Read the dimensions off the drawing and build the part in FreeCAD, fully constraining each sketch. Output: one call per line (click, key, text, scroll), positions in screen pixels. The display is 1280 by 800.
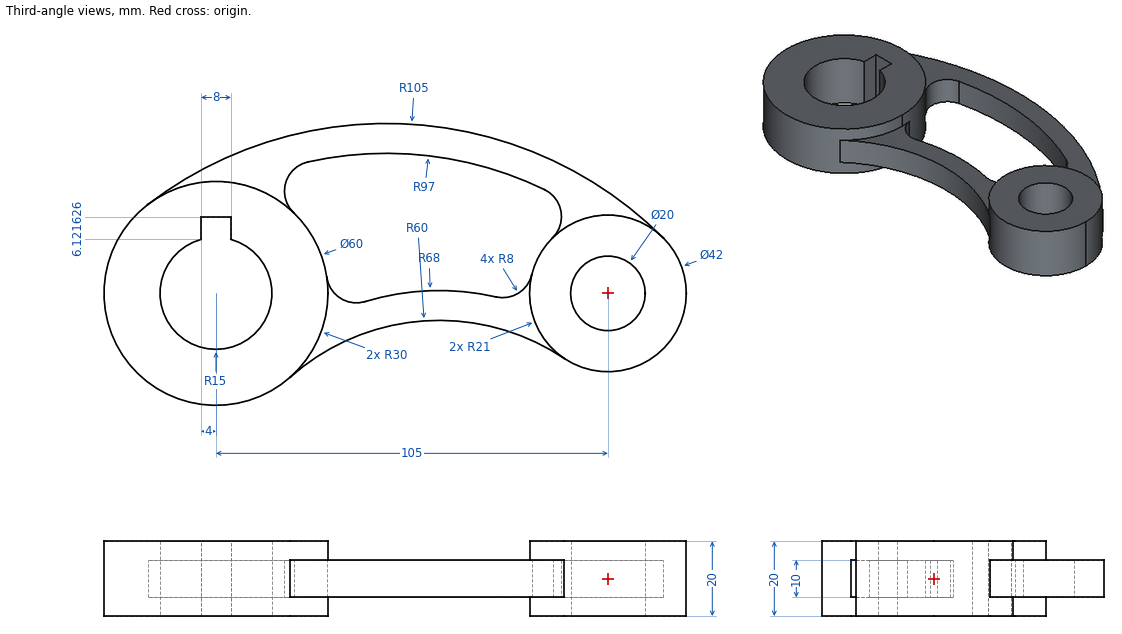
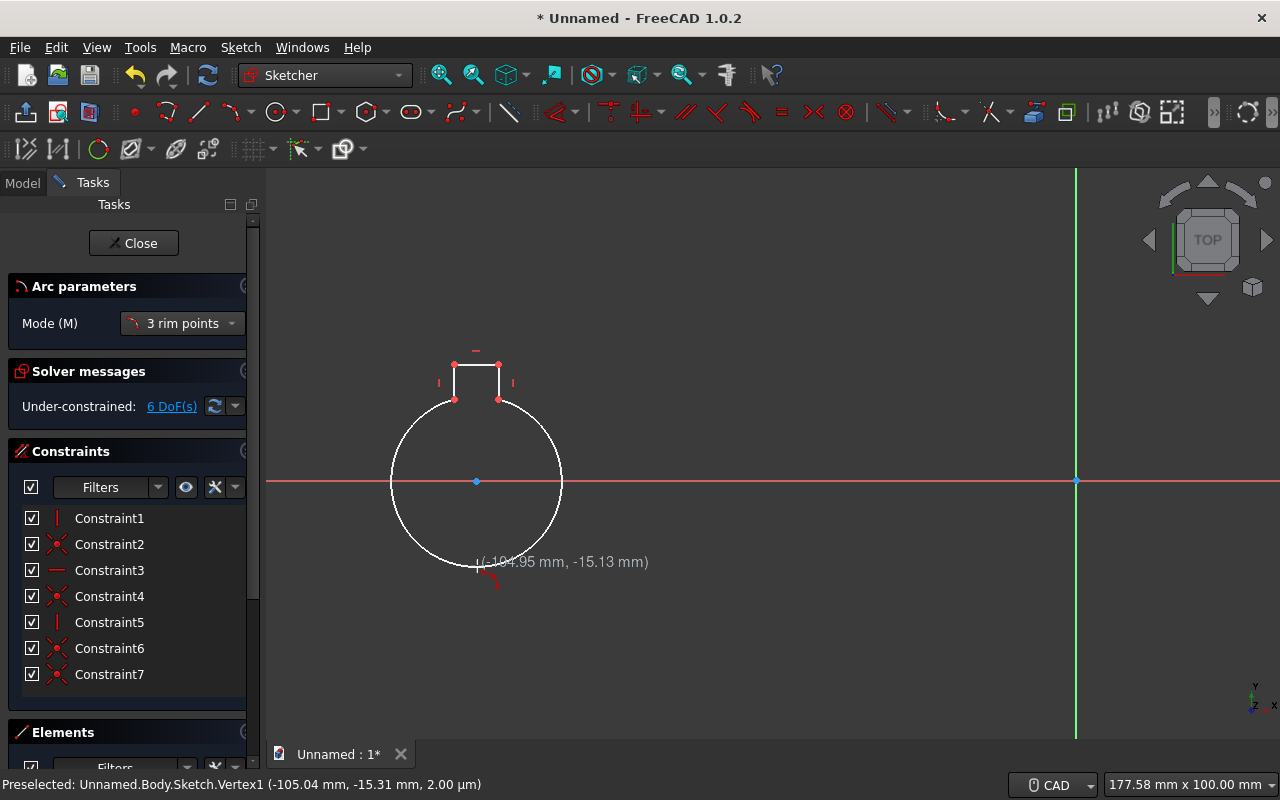
key(g)
key(c)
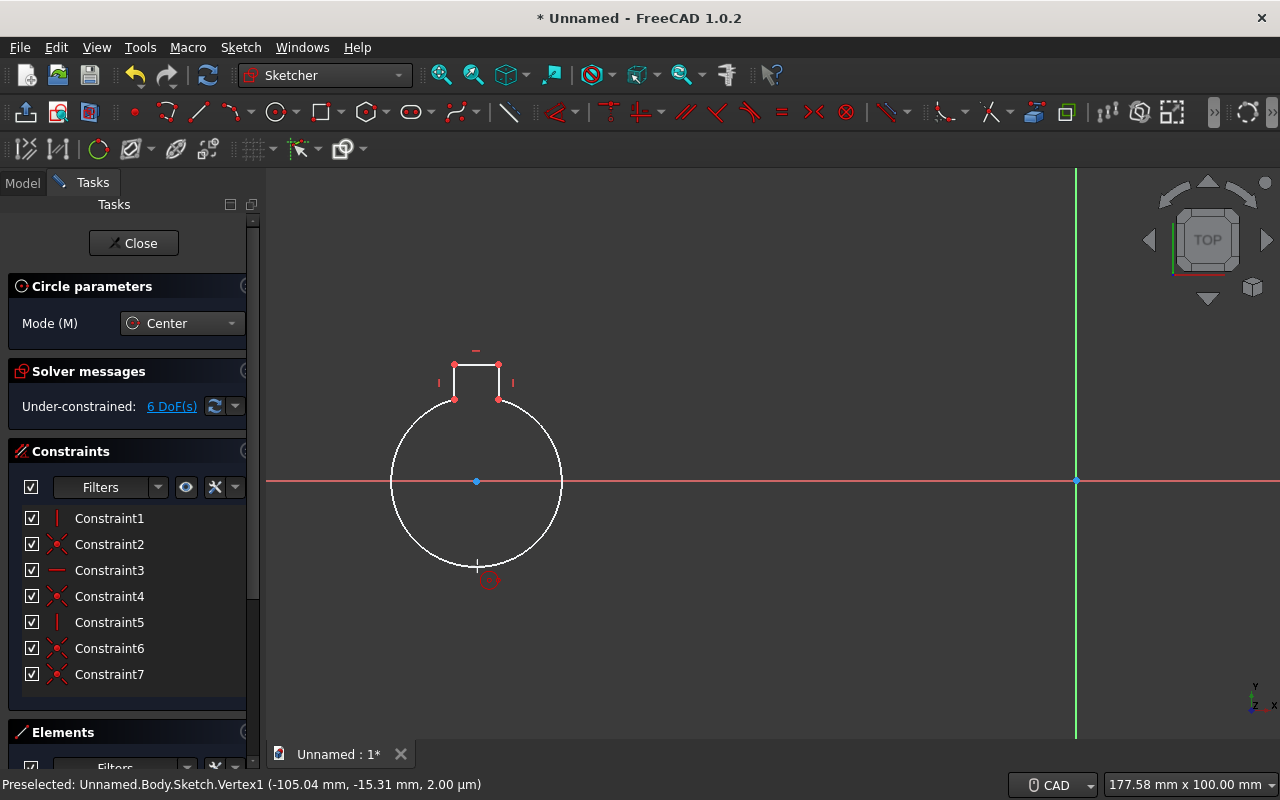
click(477, 481)
move(598, 359)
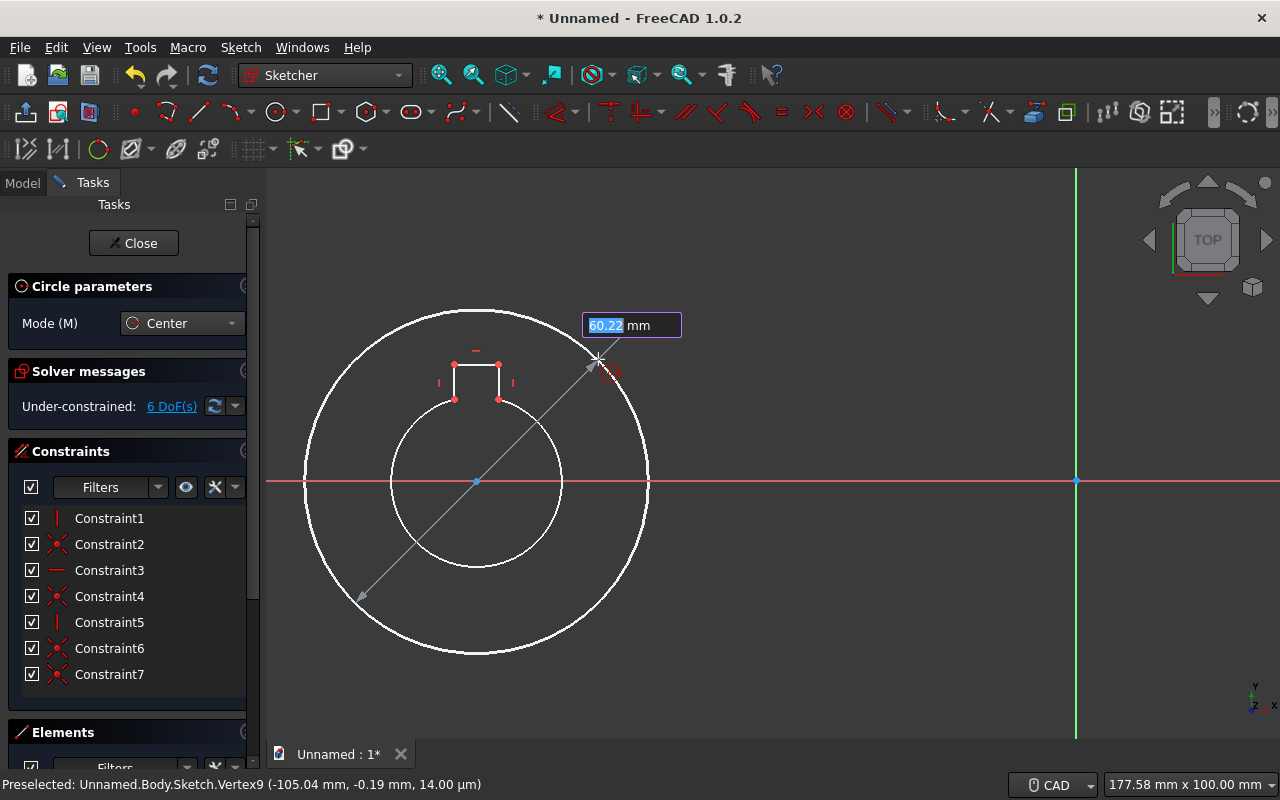
text(60)
key(Return)
key(Escape)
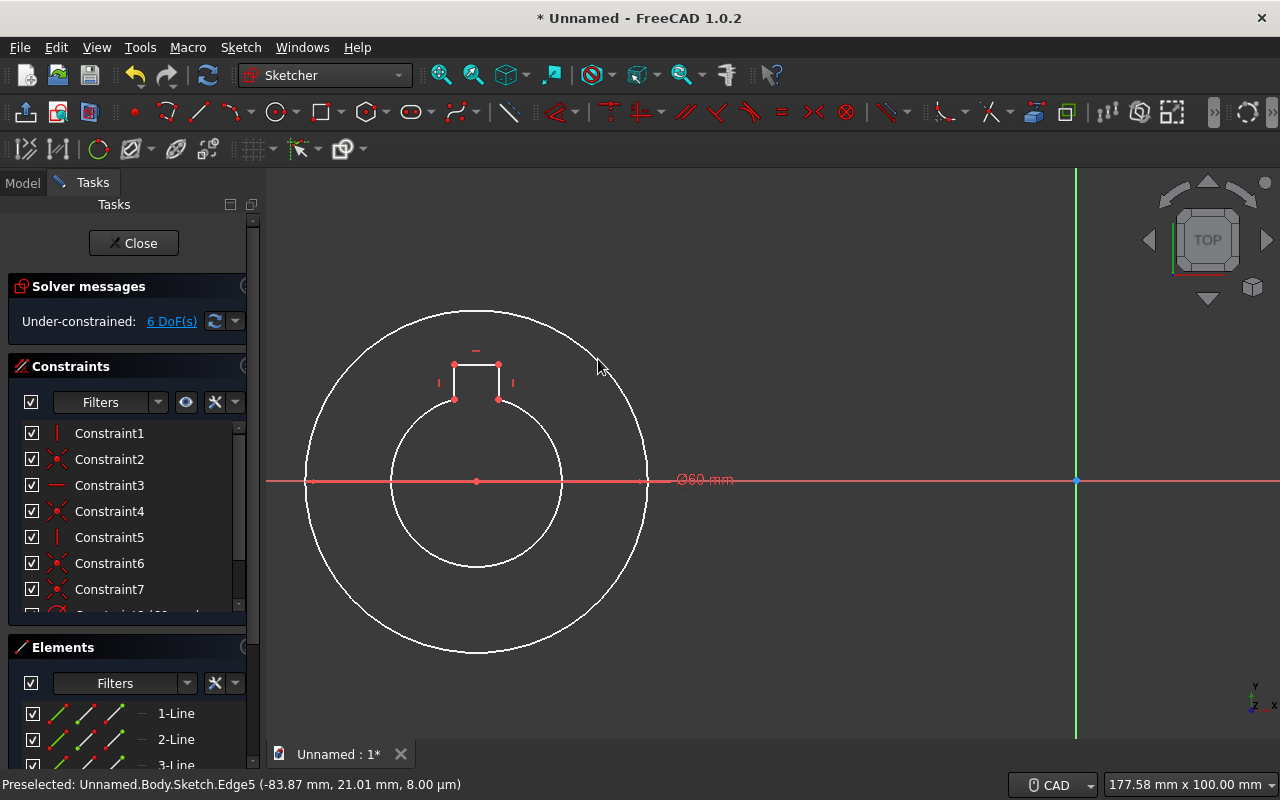
click(477, 482)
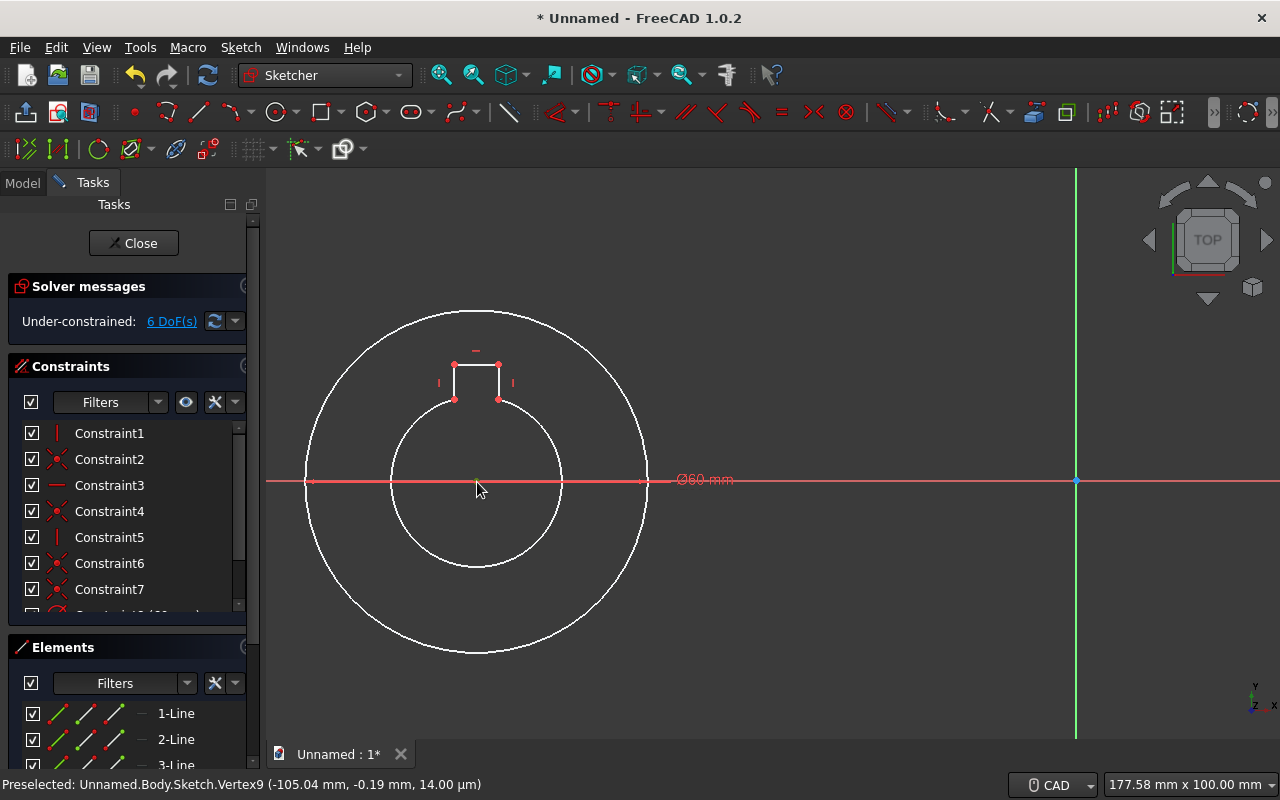
click(353, 481)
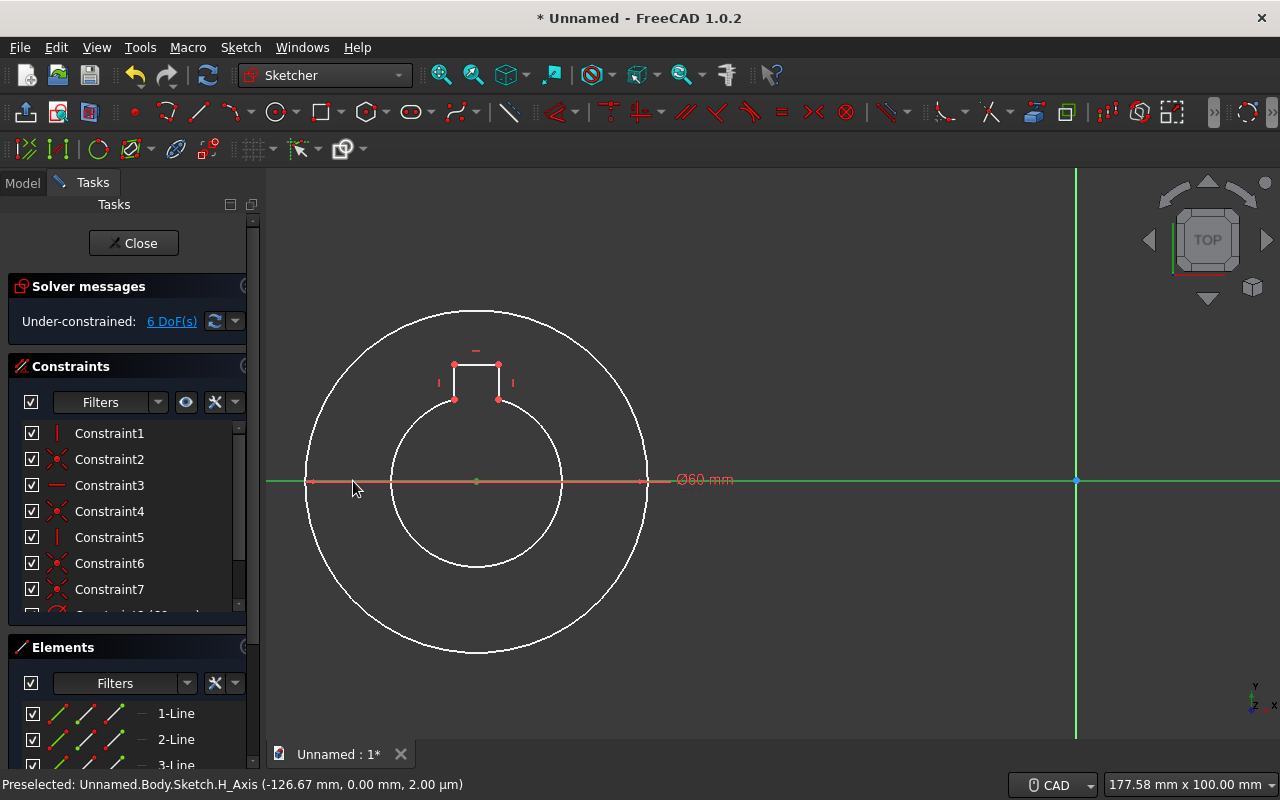
key(c)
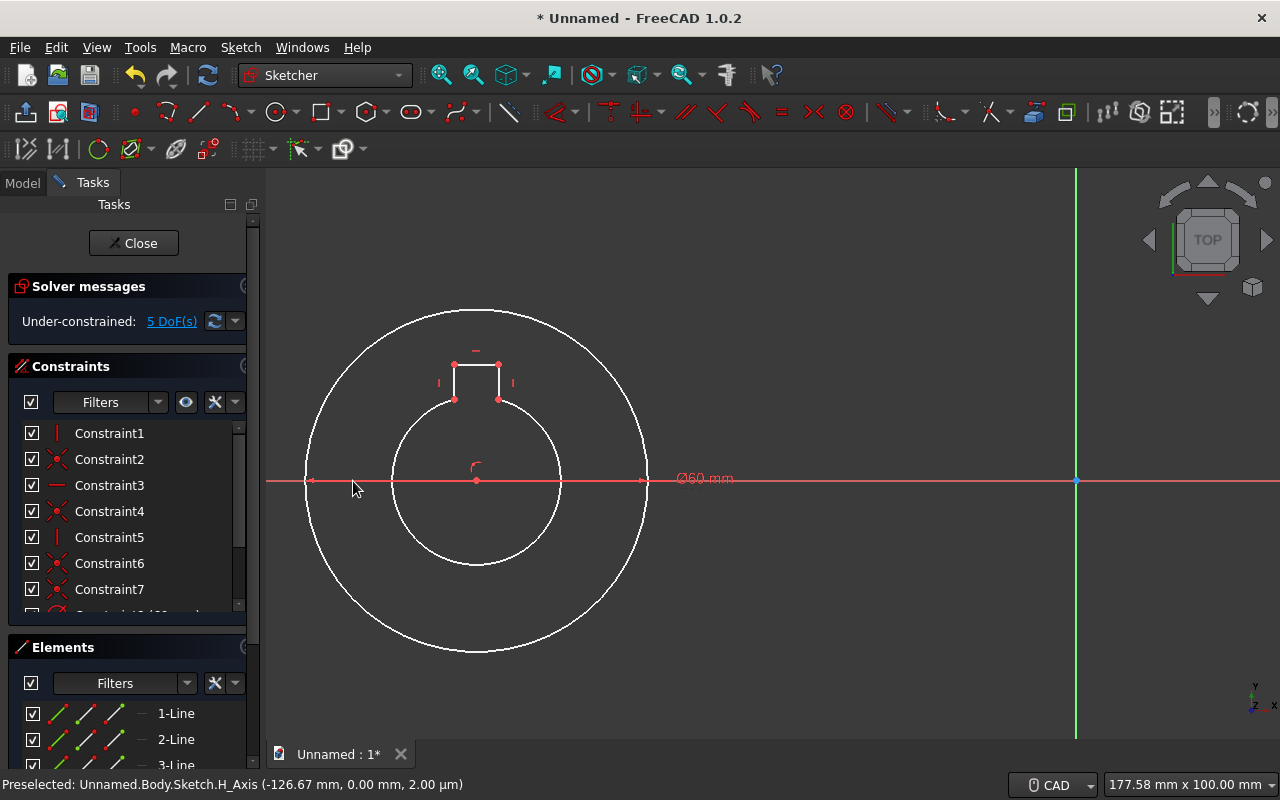
key(d)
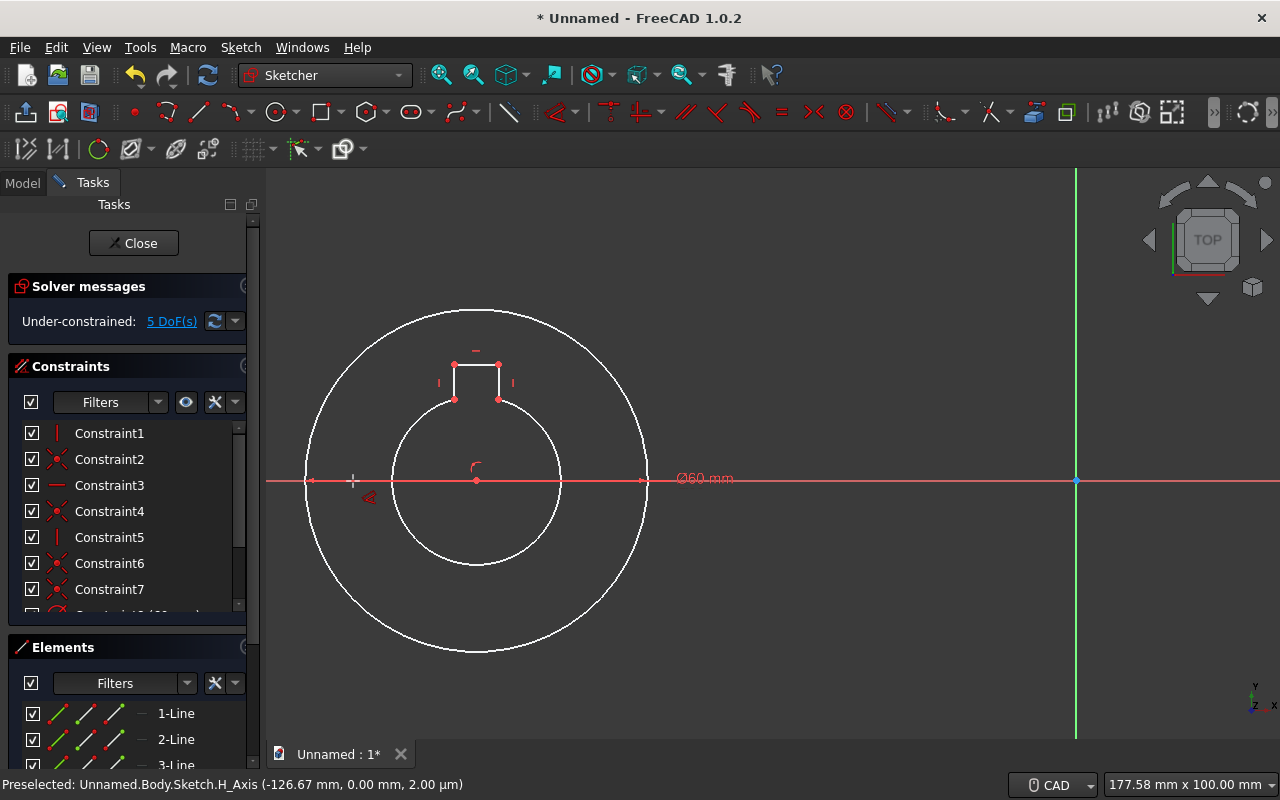
click(400, 515)
click(371, 528)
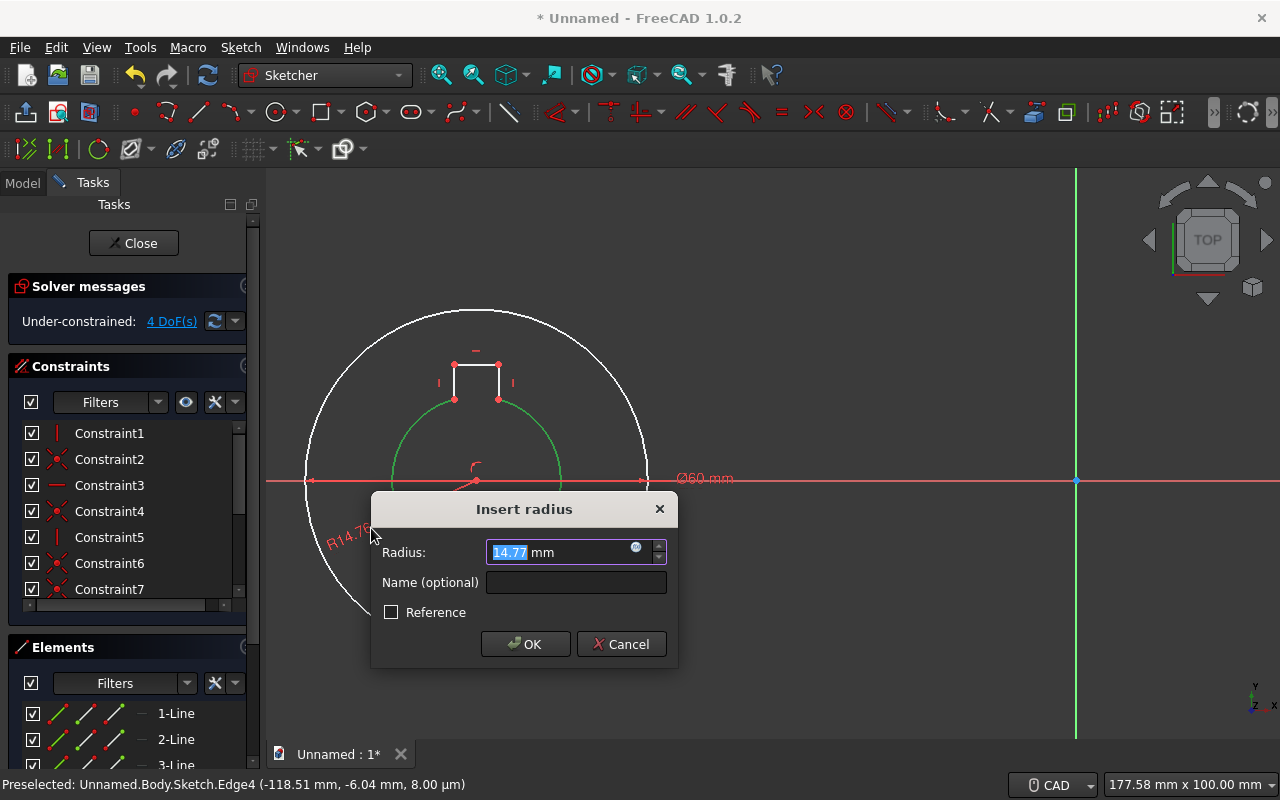
text(15)
key(Return)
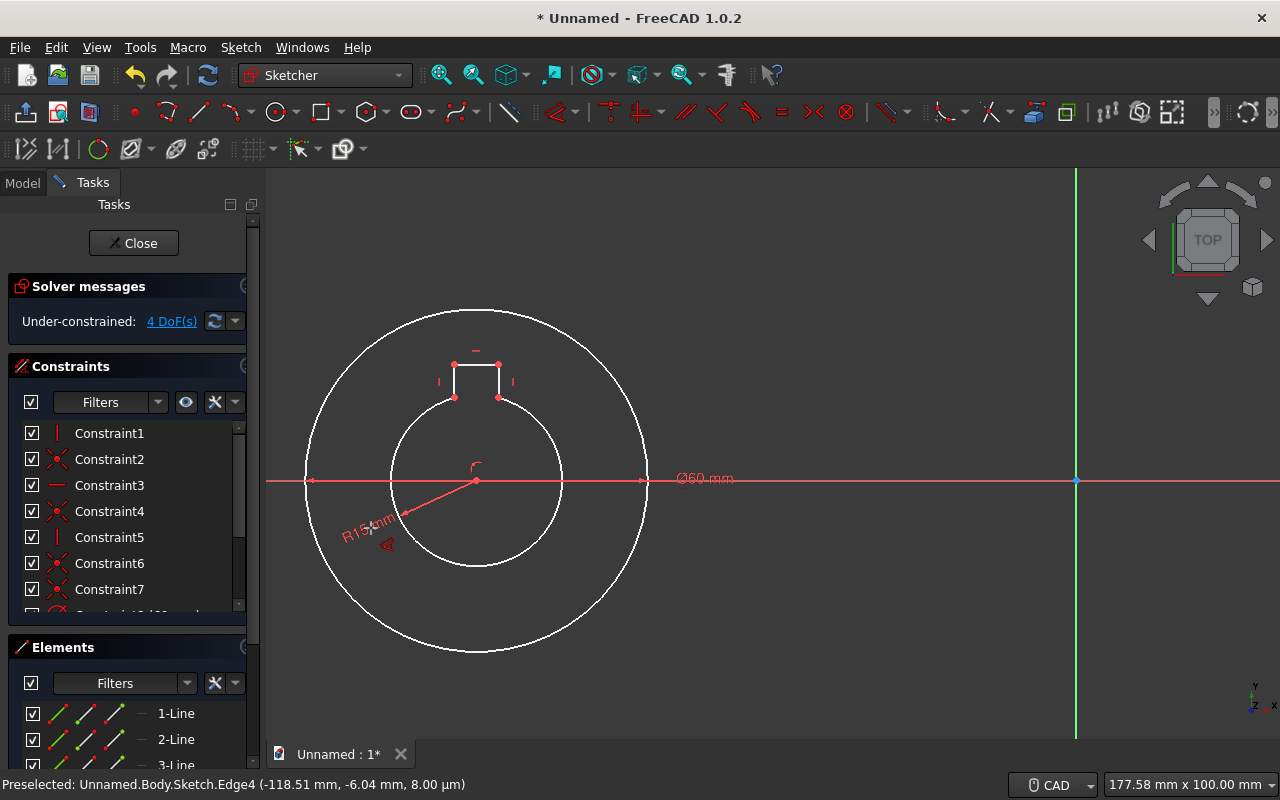
click(468, 365)
click(477, 331)